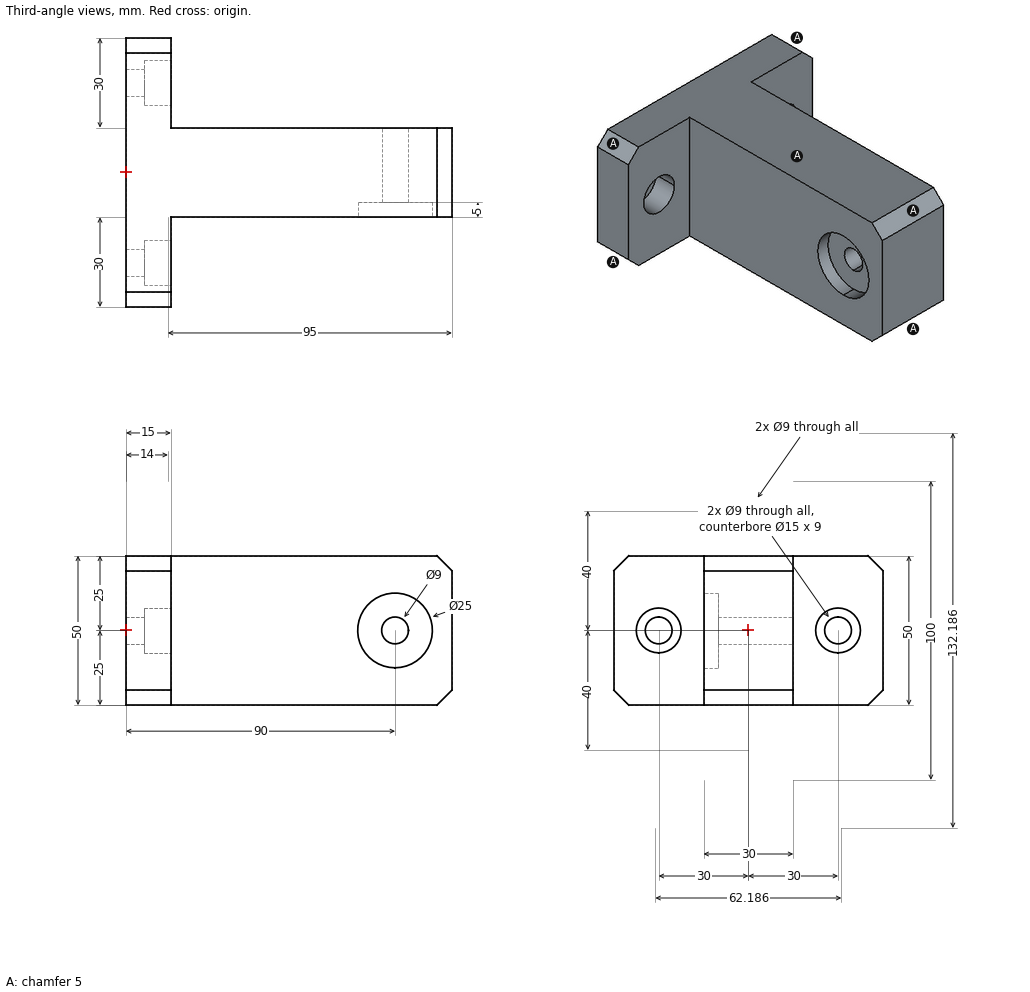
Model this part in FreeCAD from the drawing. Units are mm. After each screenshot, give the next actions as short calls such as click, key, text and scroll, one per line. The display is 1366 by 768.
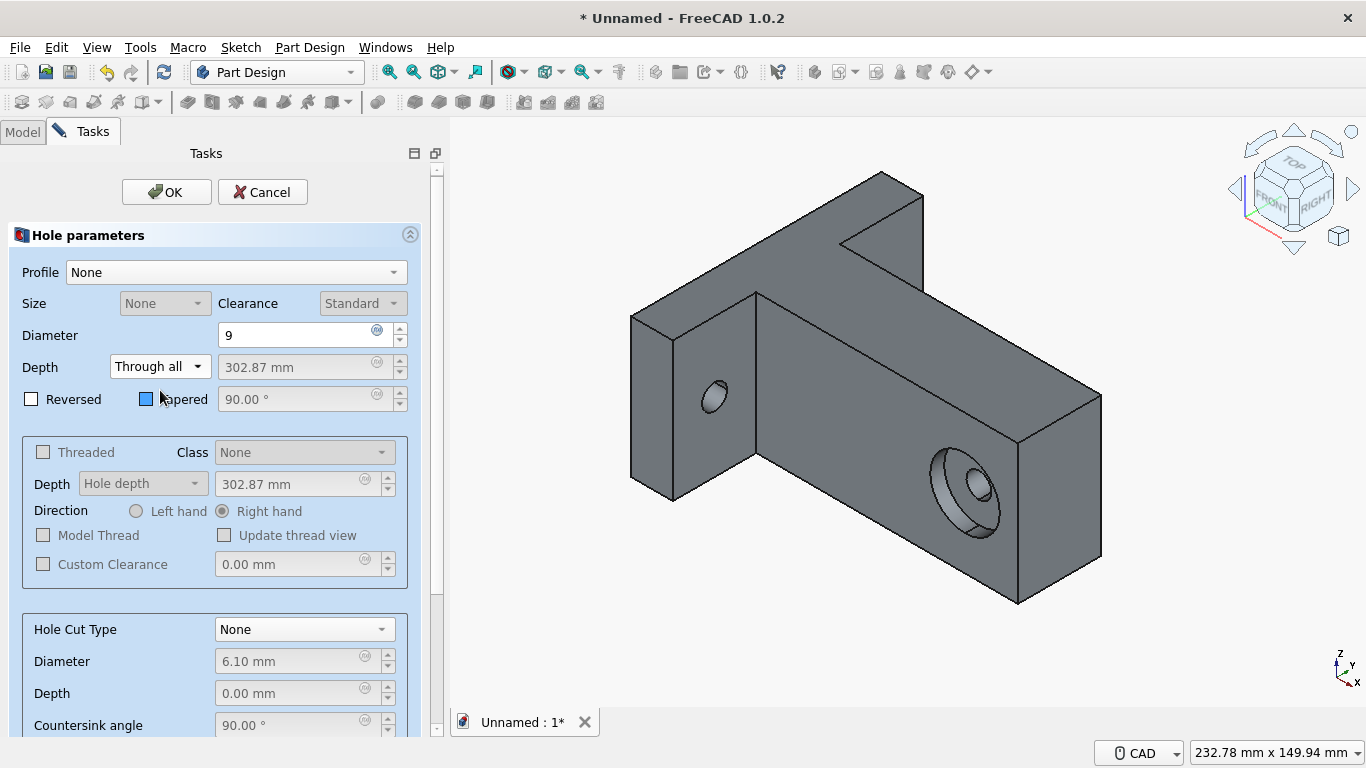
click(306, 630)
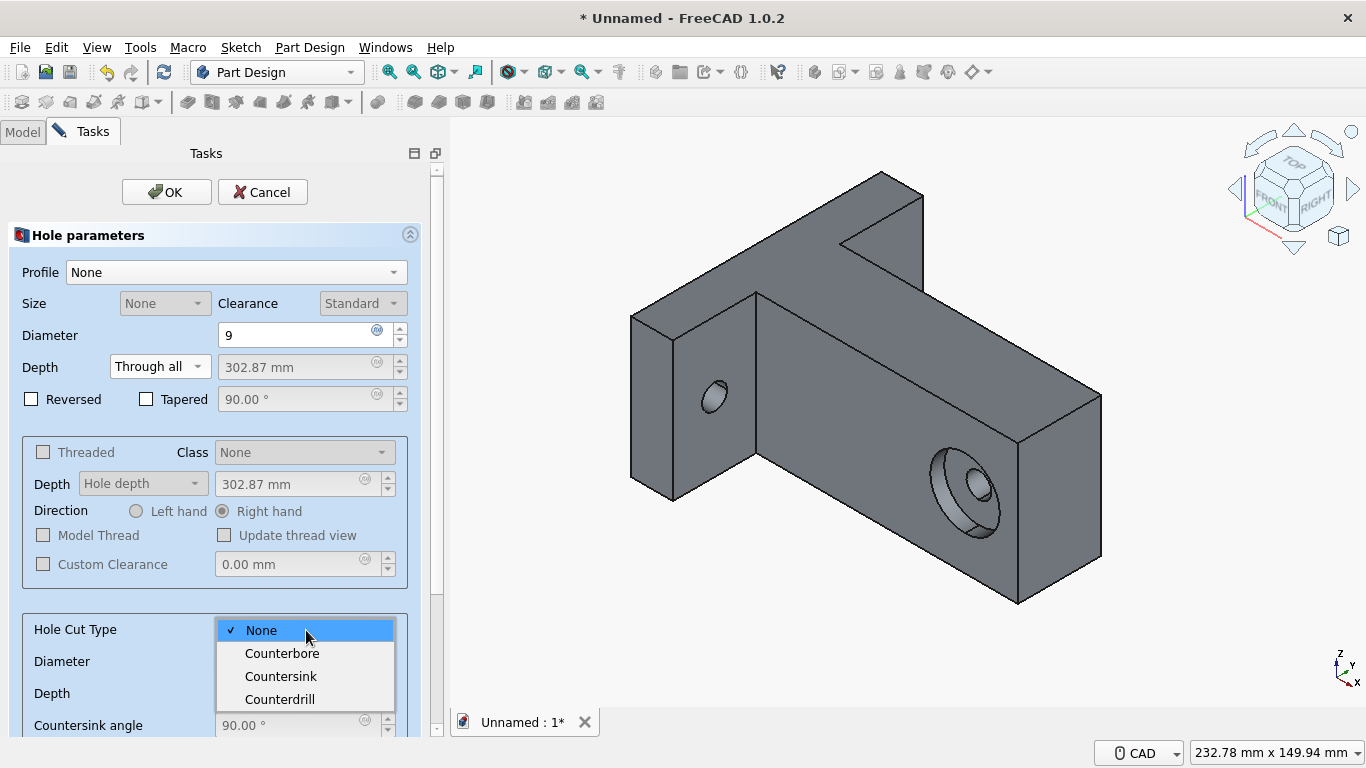
click(304, 654)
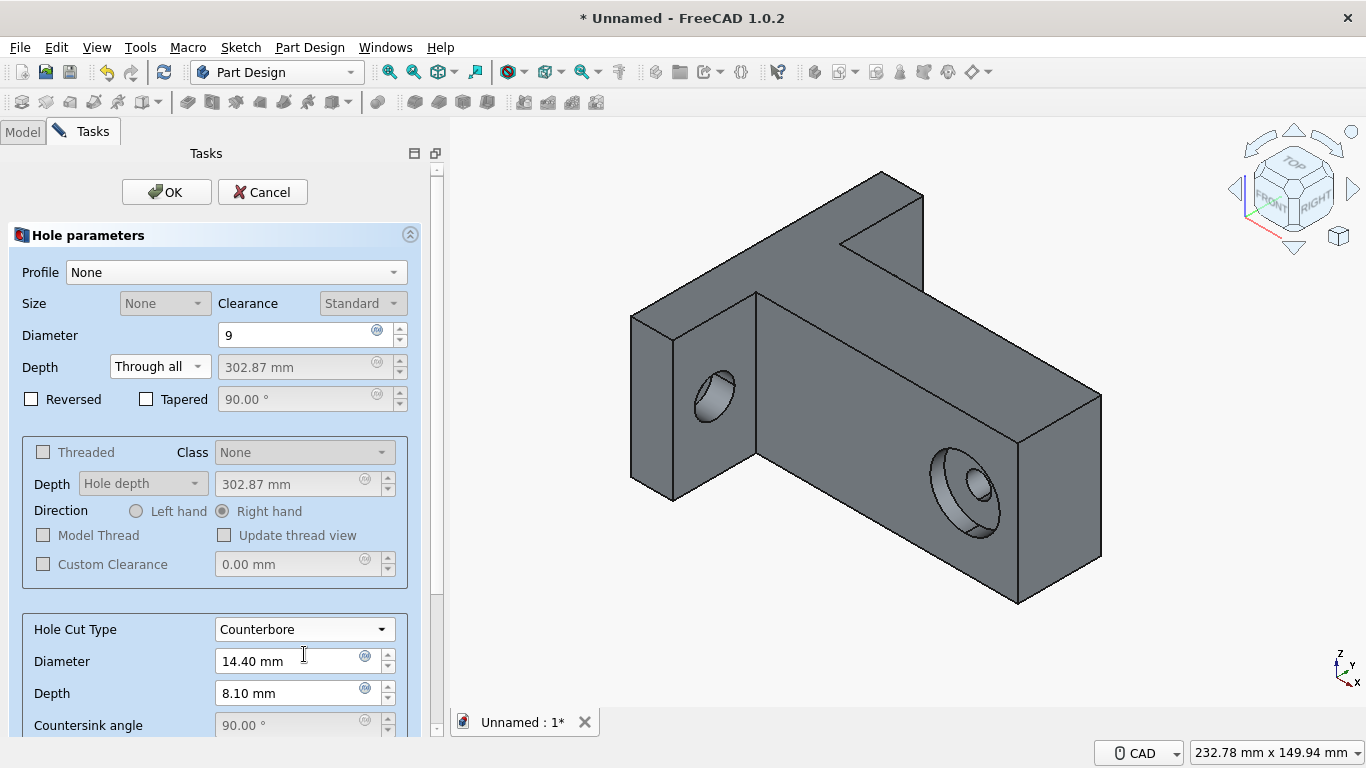
triple_click(298, 661)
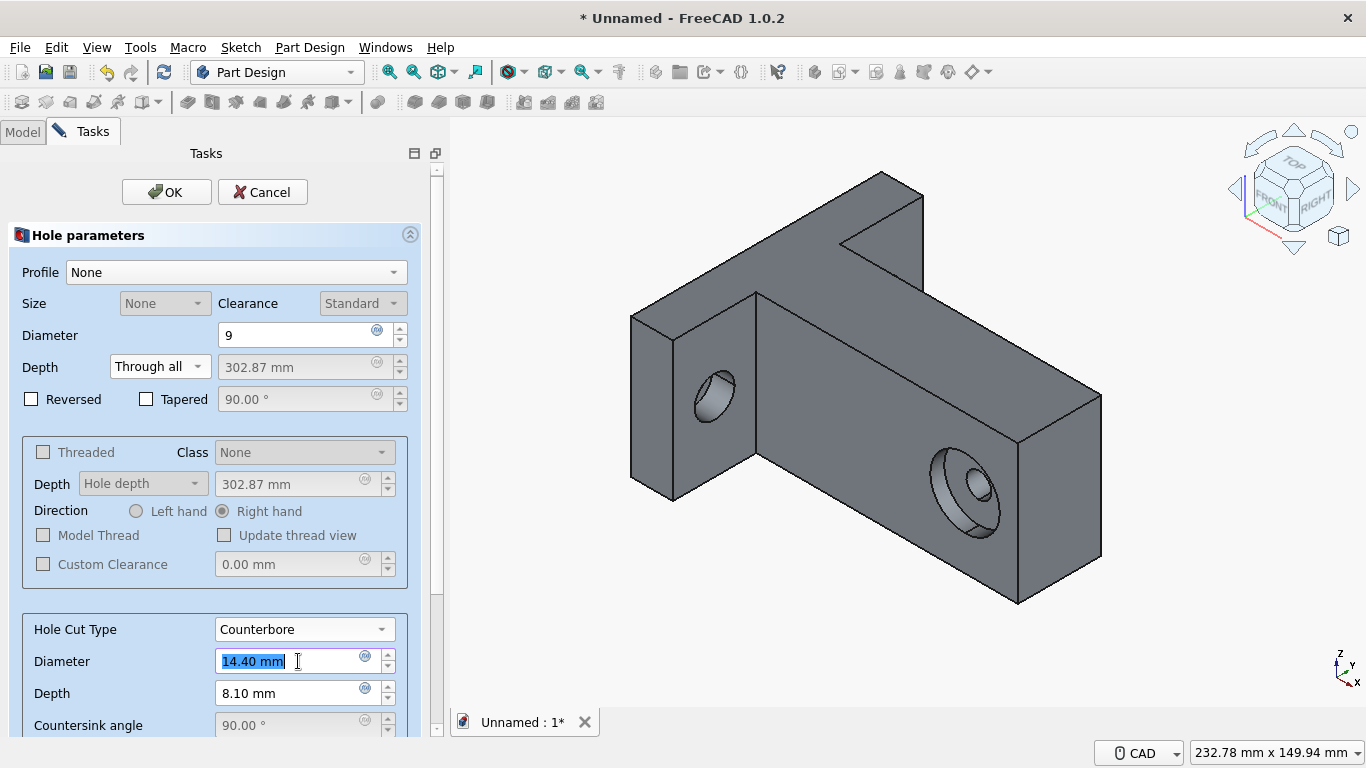
text(15)
key(Tab)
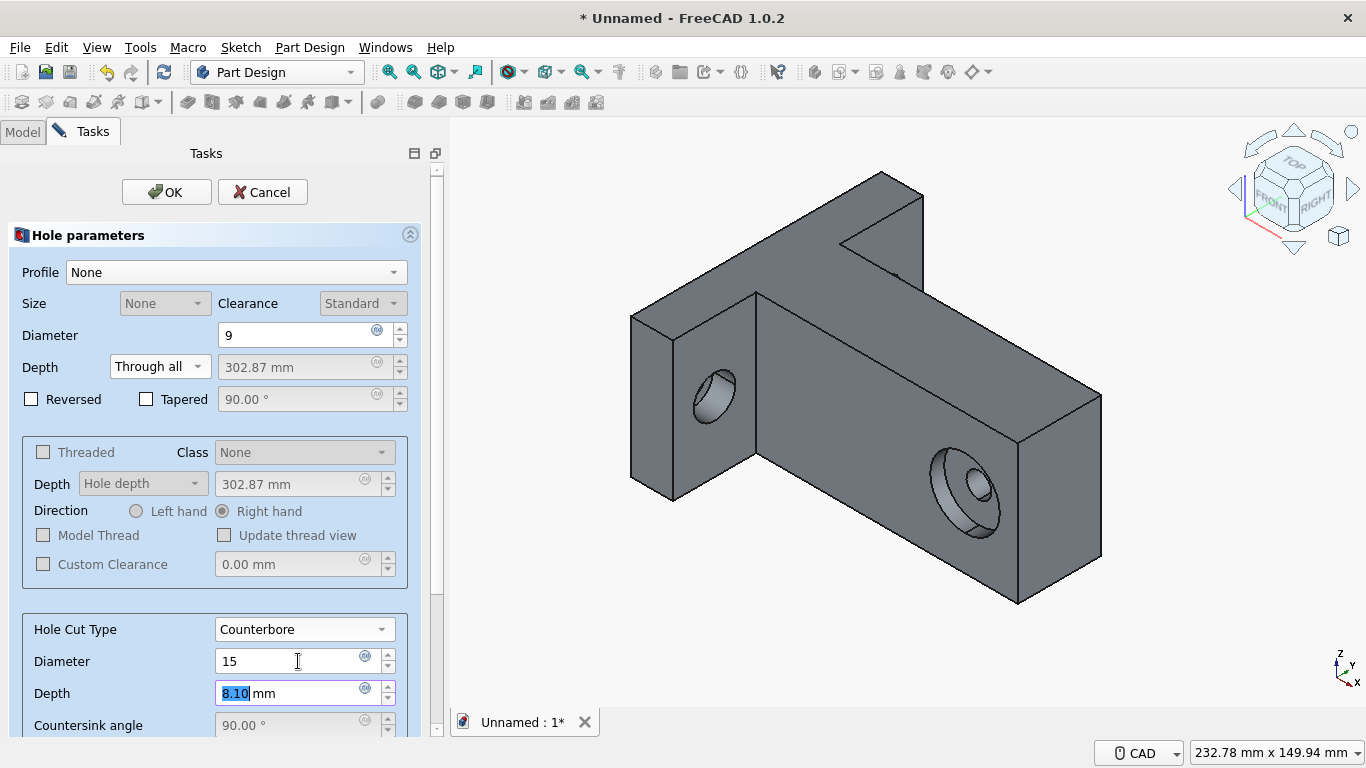
text(9)
key(Tab)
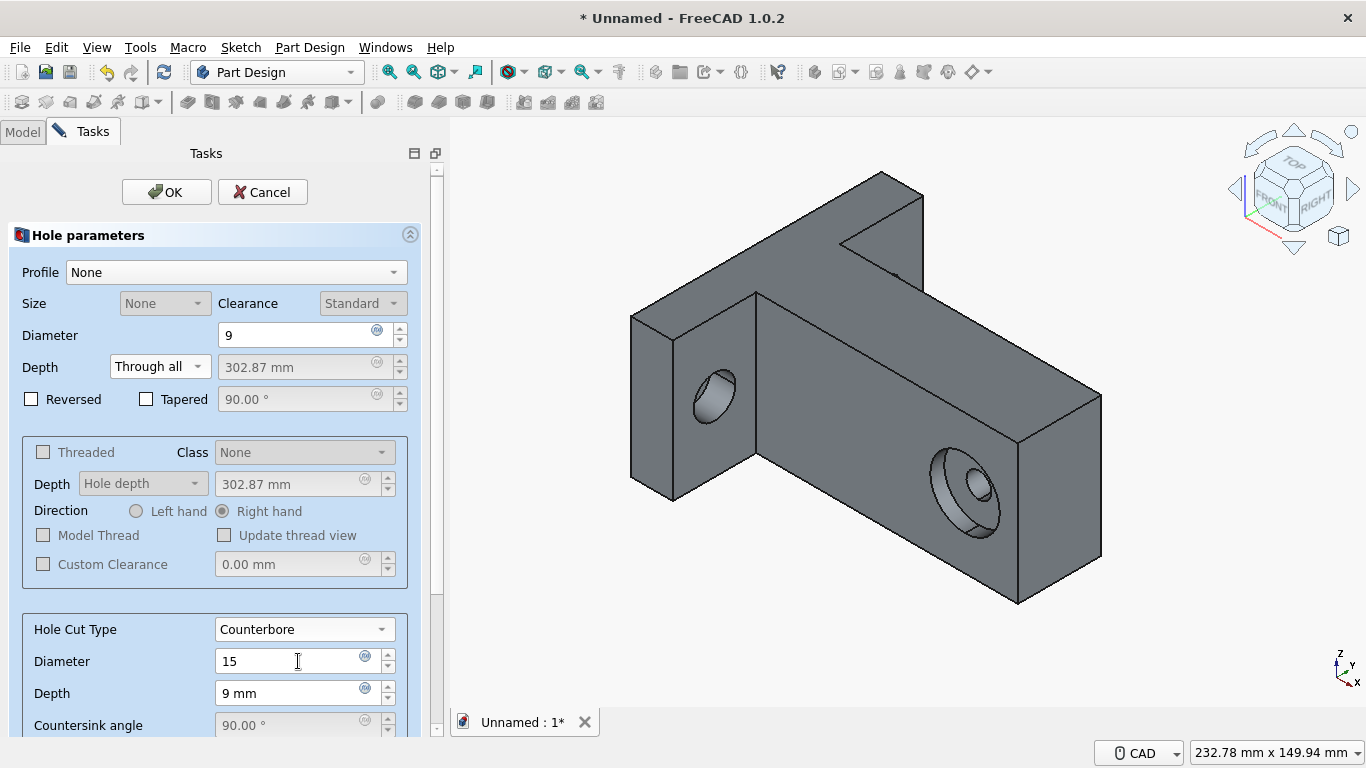
click(167, 192)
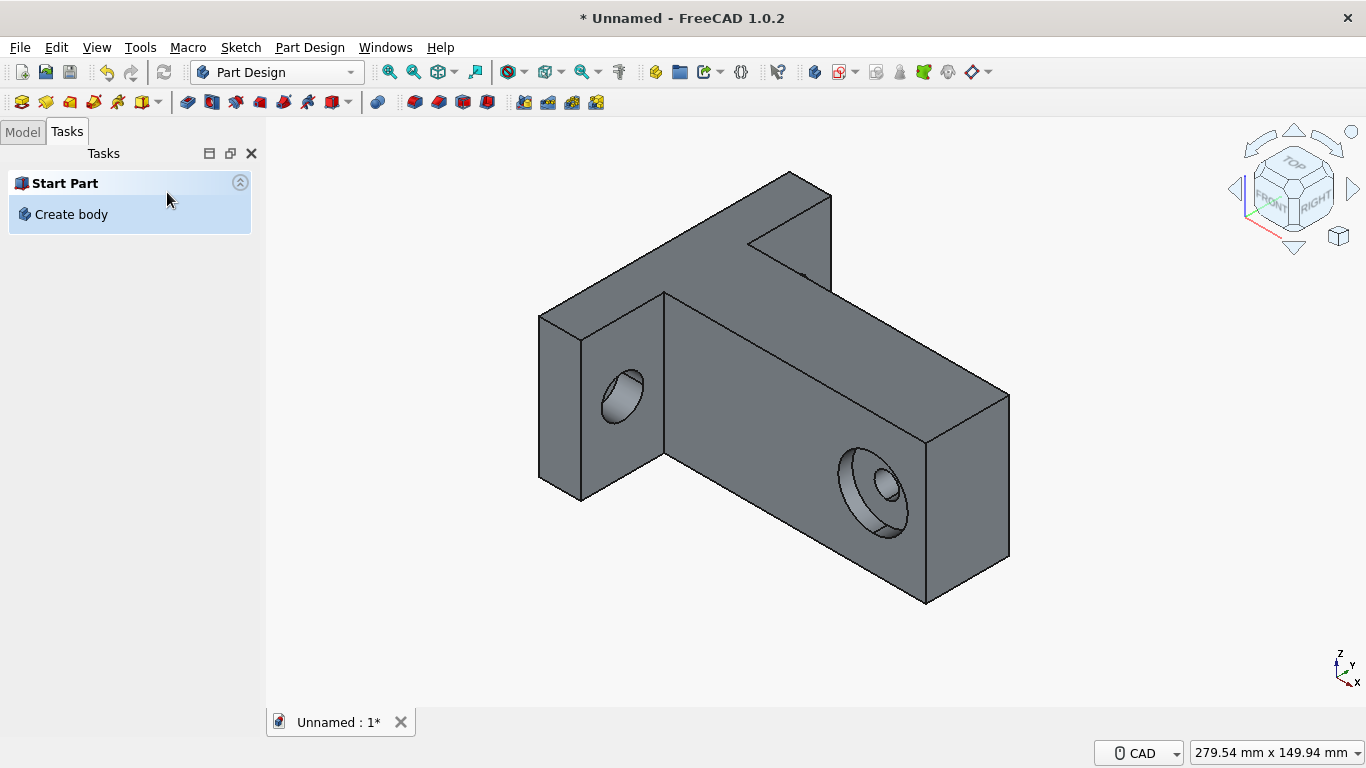
click(968, 418)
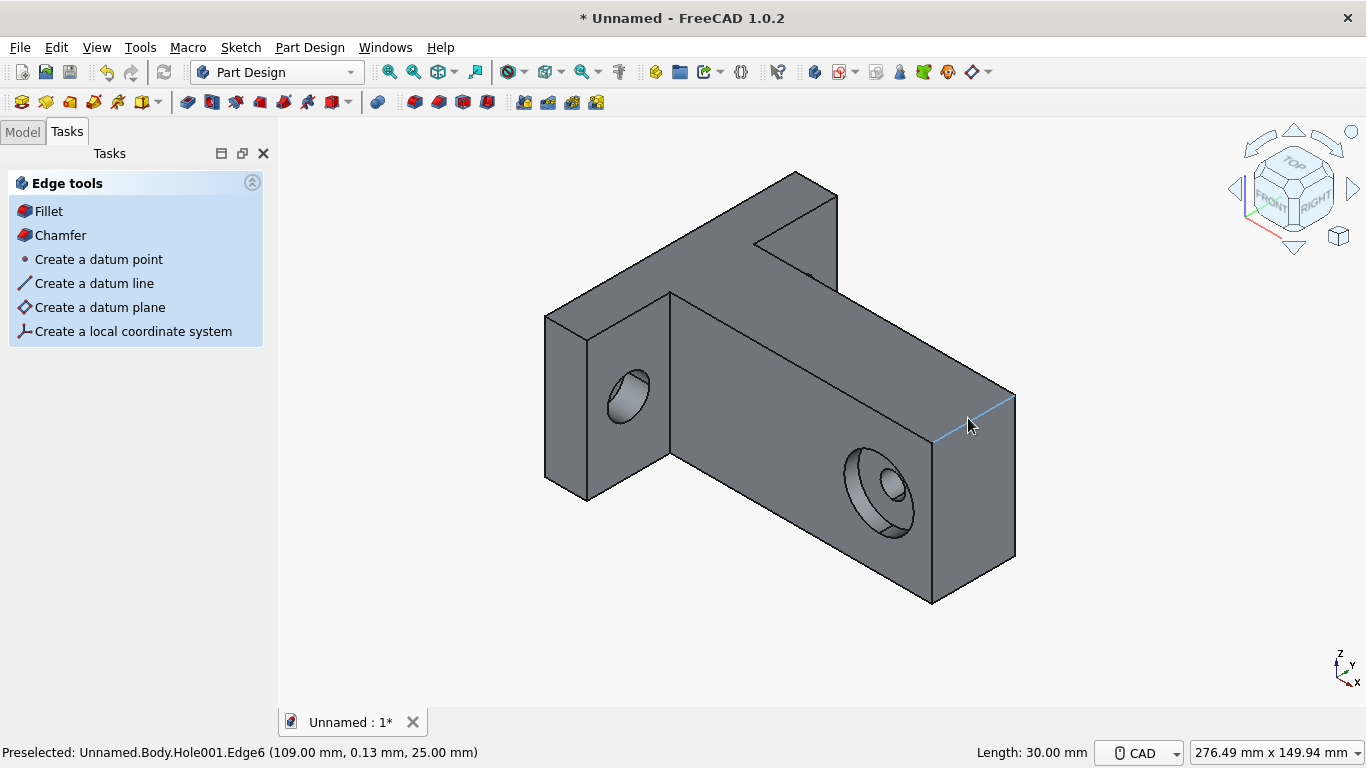
click(566, 327, ctrl)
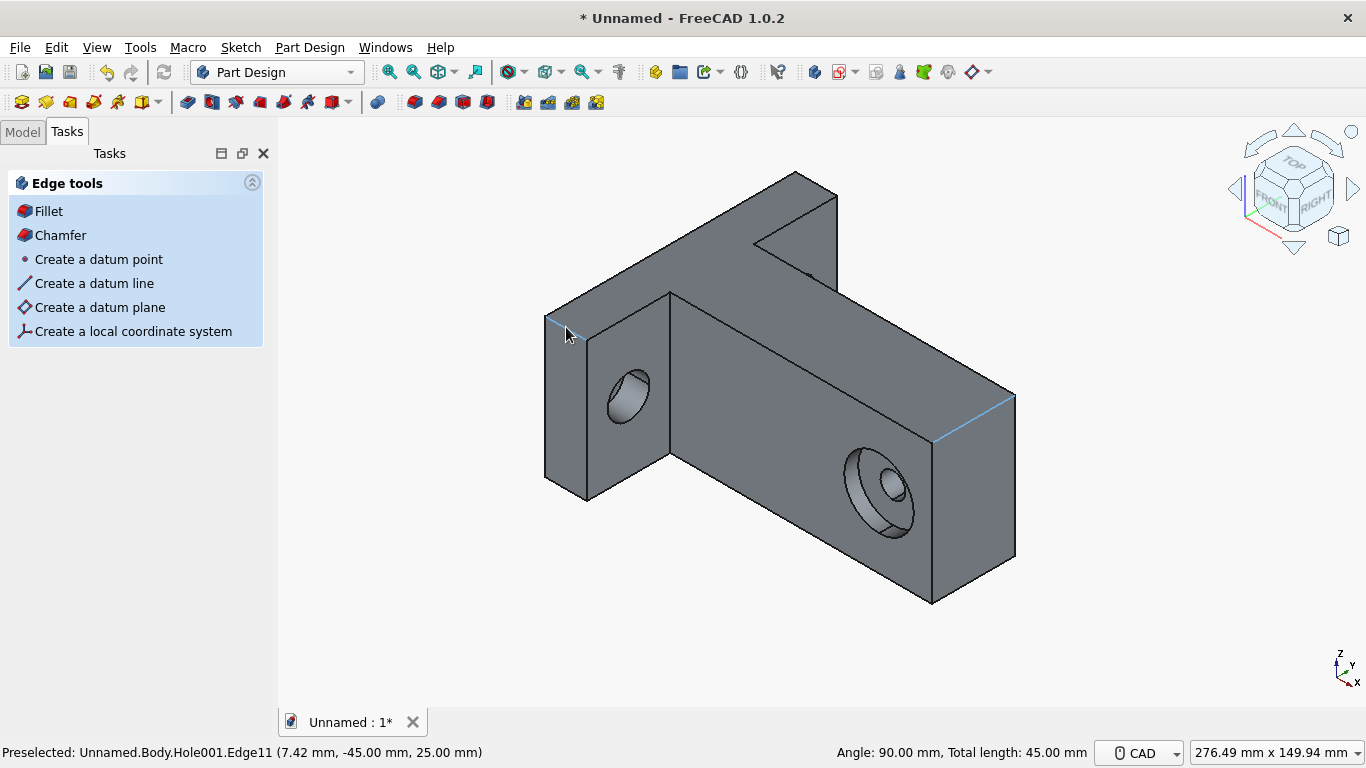
key(2)